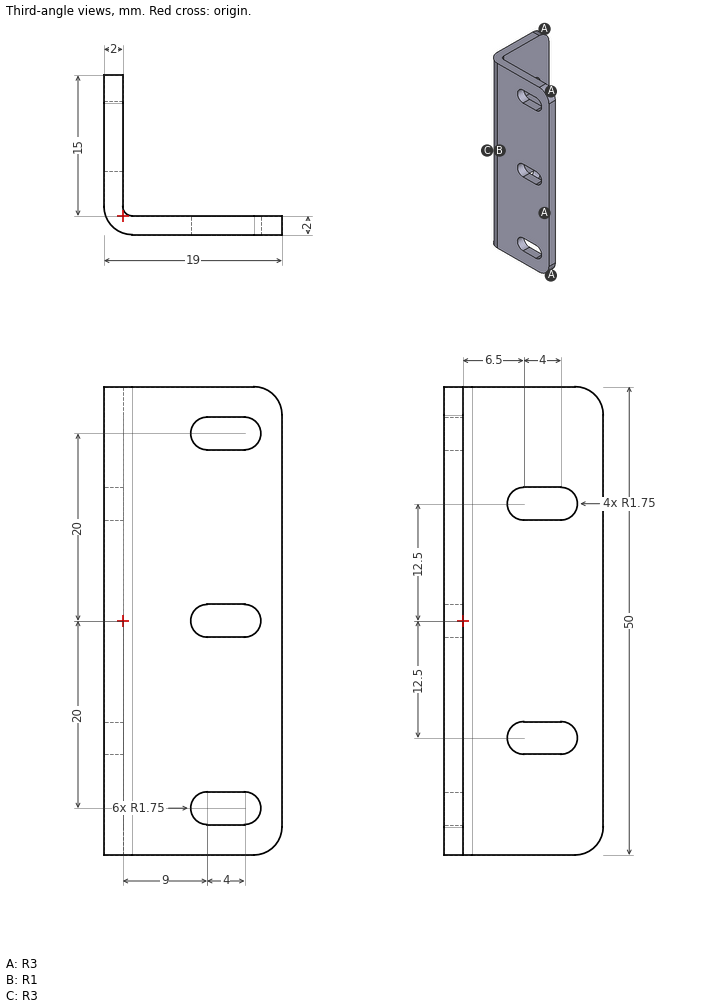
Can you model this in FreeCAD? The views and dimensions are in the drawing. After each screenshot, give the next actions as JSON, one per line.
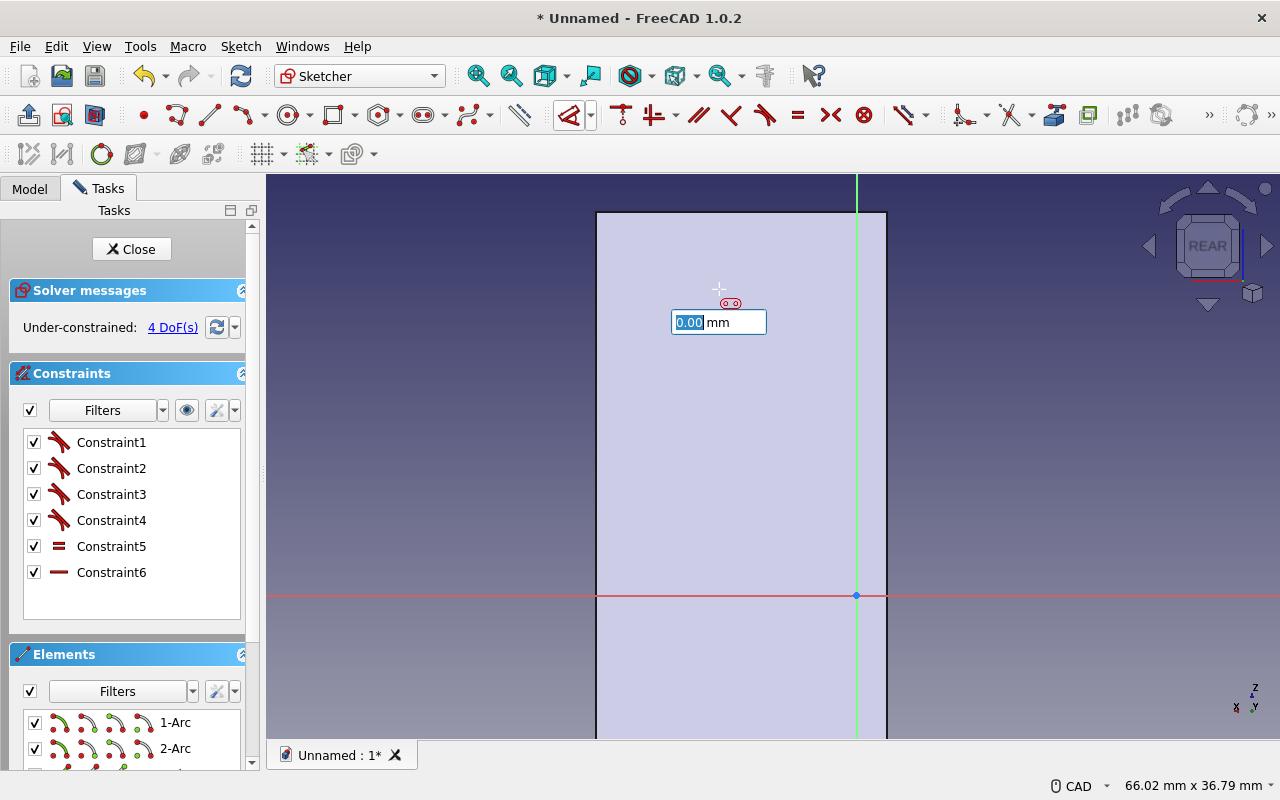
{"action": "left_click", "coordinate": [688, 262]}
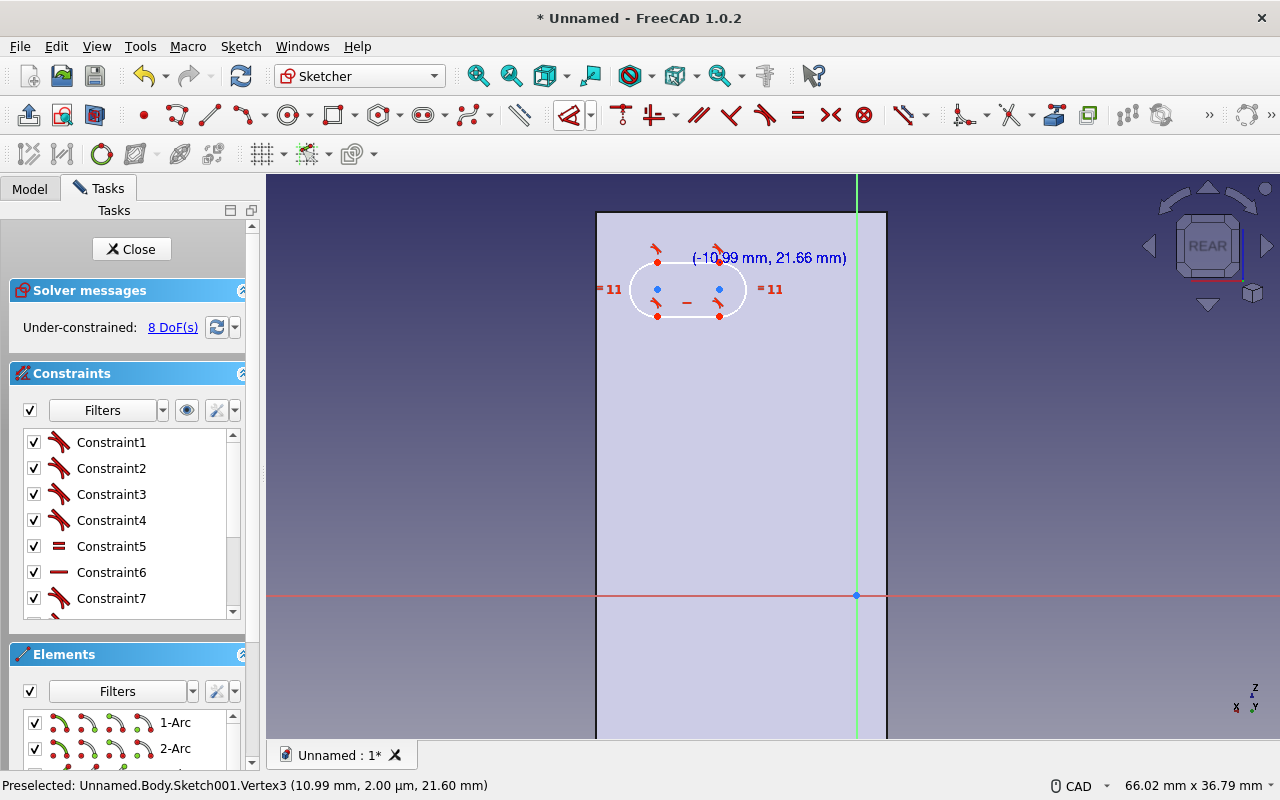
{"action": "left_click", "coordinate": [657, 596]}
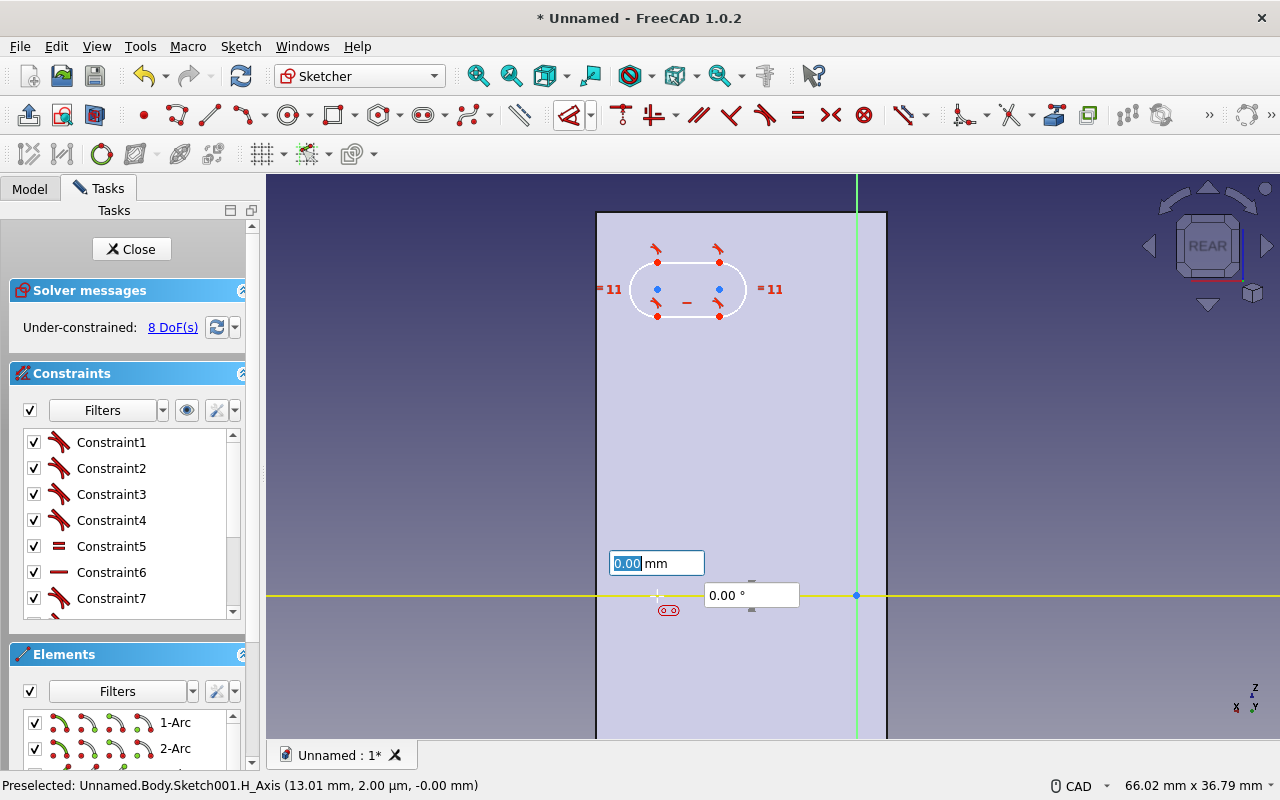
{"action": "left_click", "coordinate": [719, 587]}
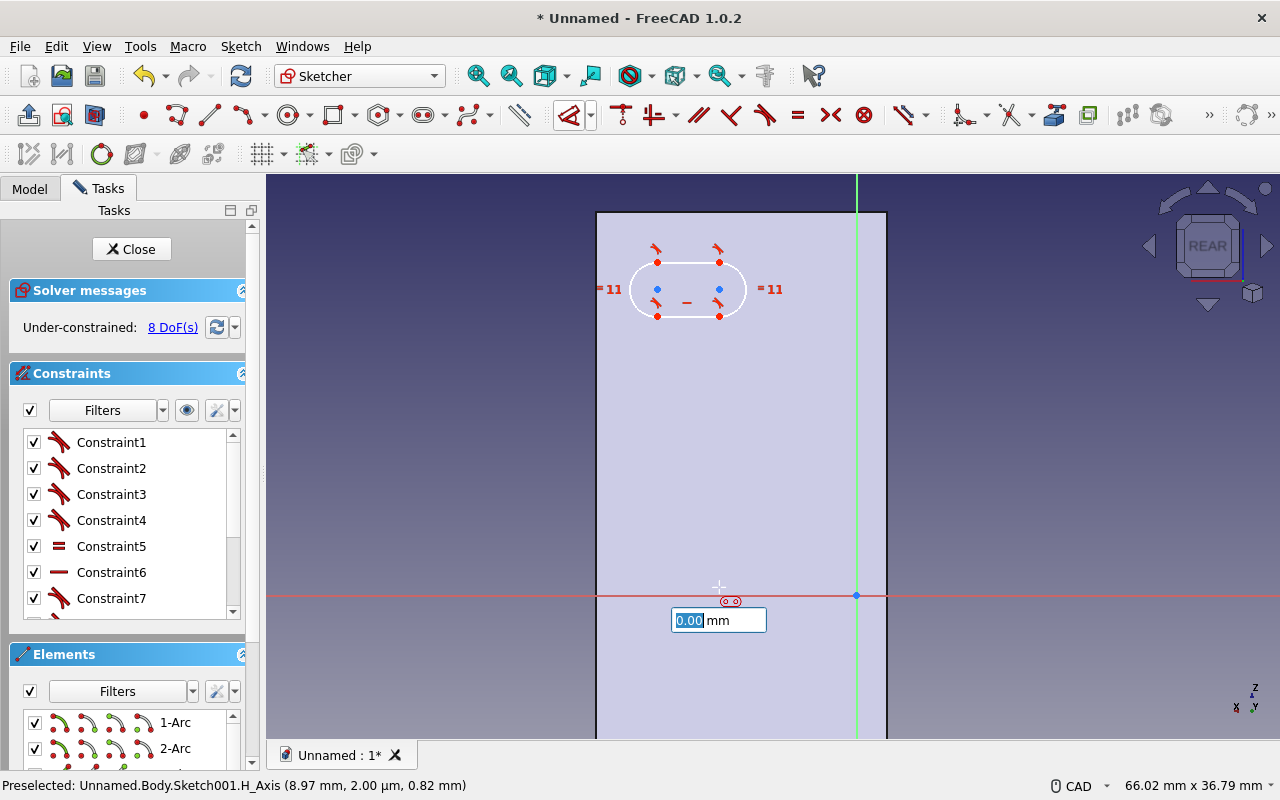
{"action": "left_click", "coordinate": [688, 623]}
{"action": "key", "text": "Escape"}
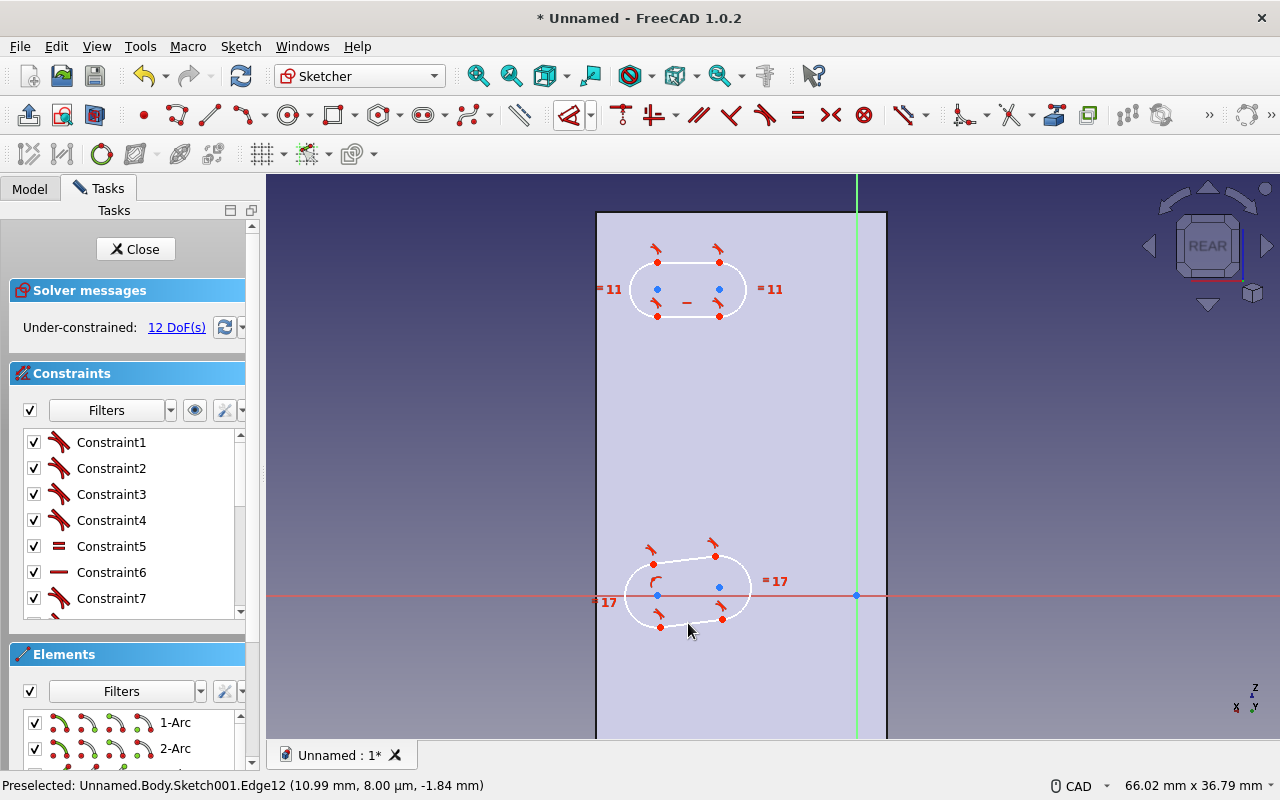
{"action": "left_click", "coordinate": [672, 562]}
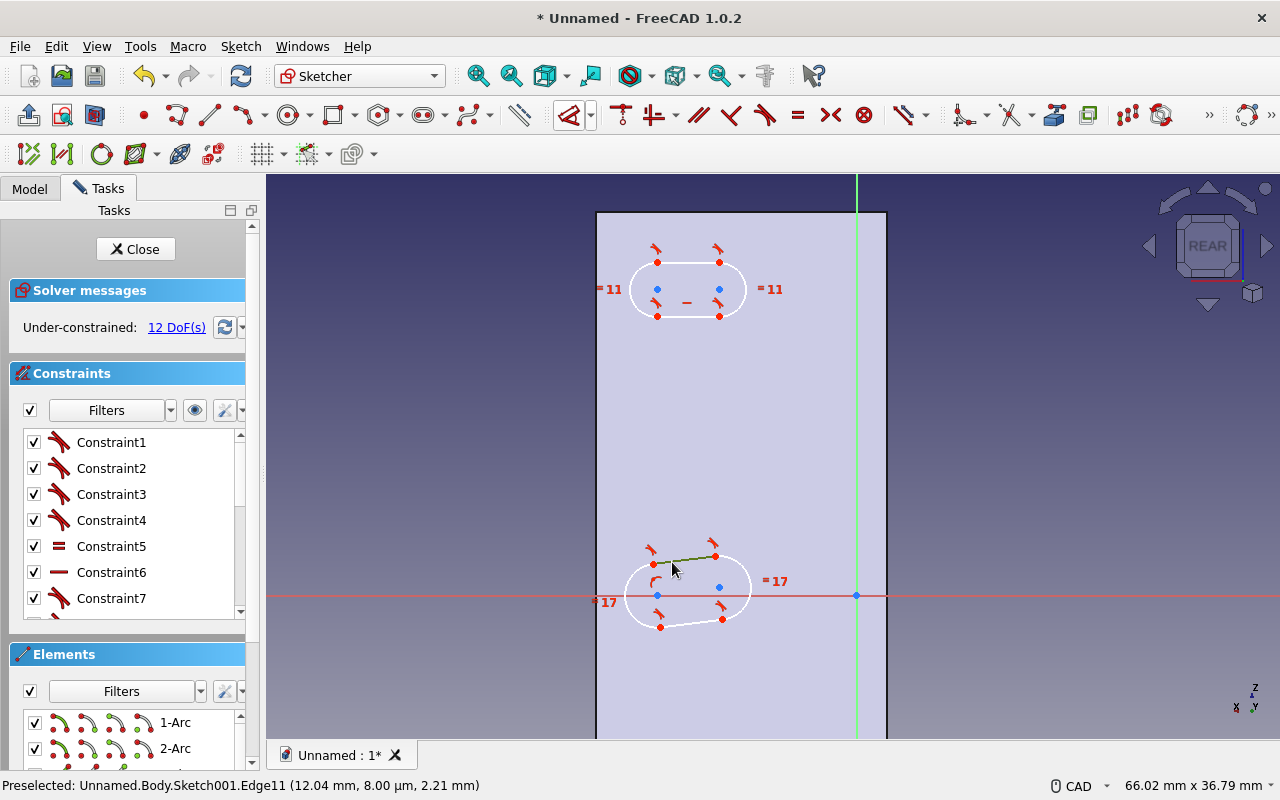
{"action": "left_click", "coordinate": [676, 116]}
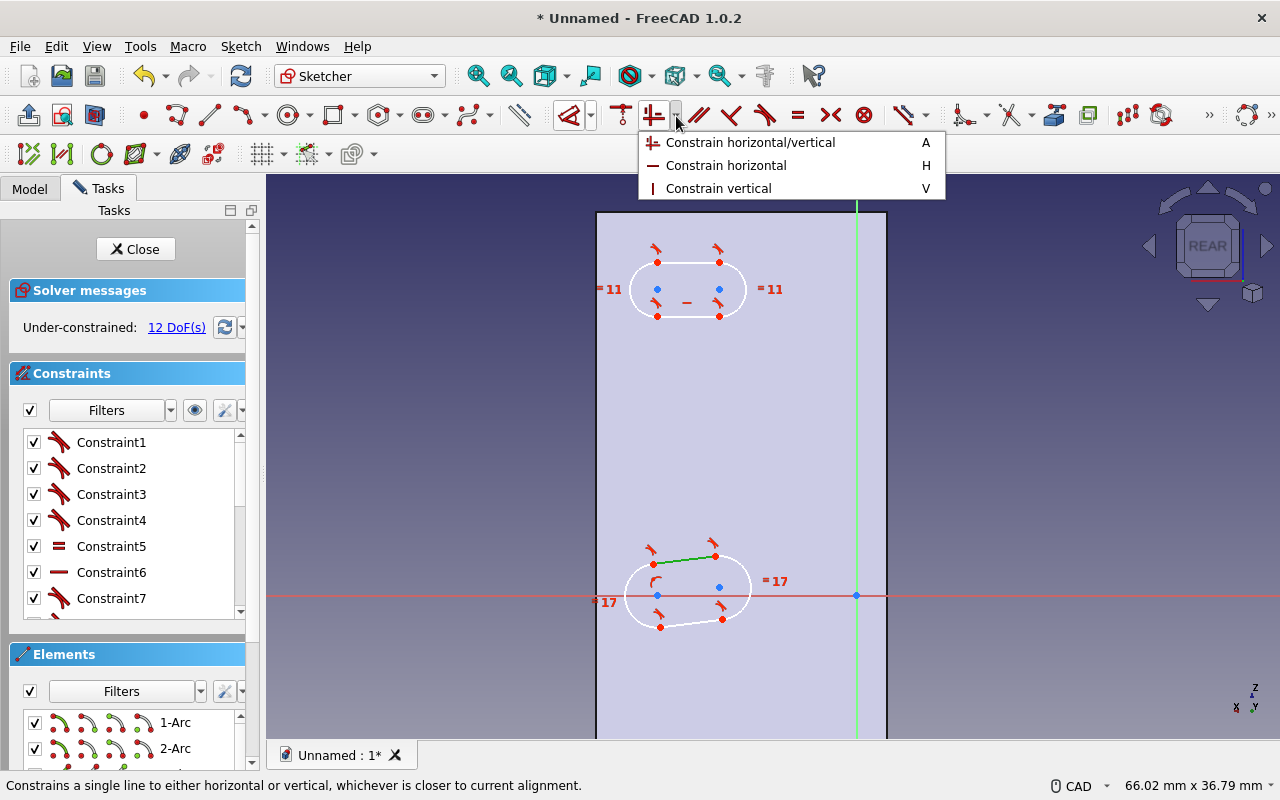
{"action": "left_click", "coordinate": [792, 166]}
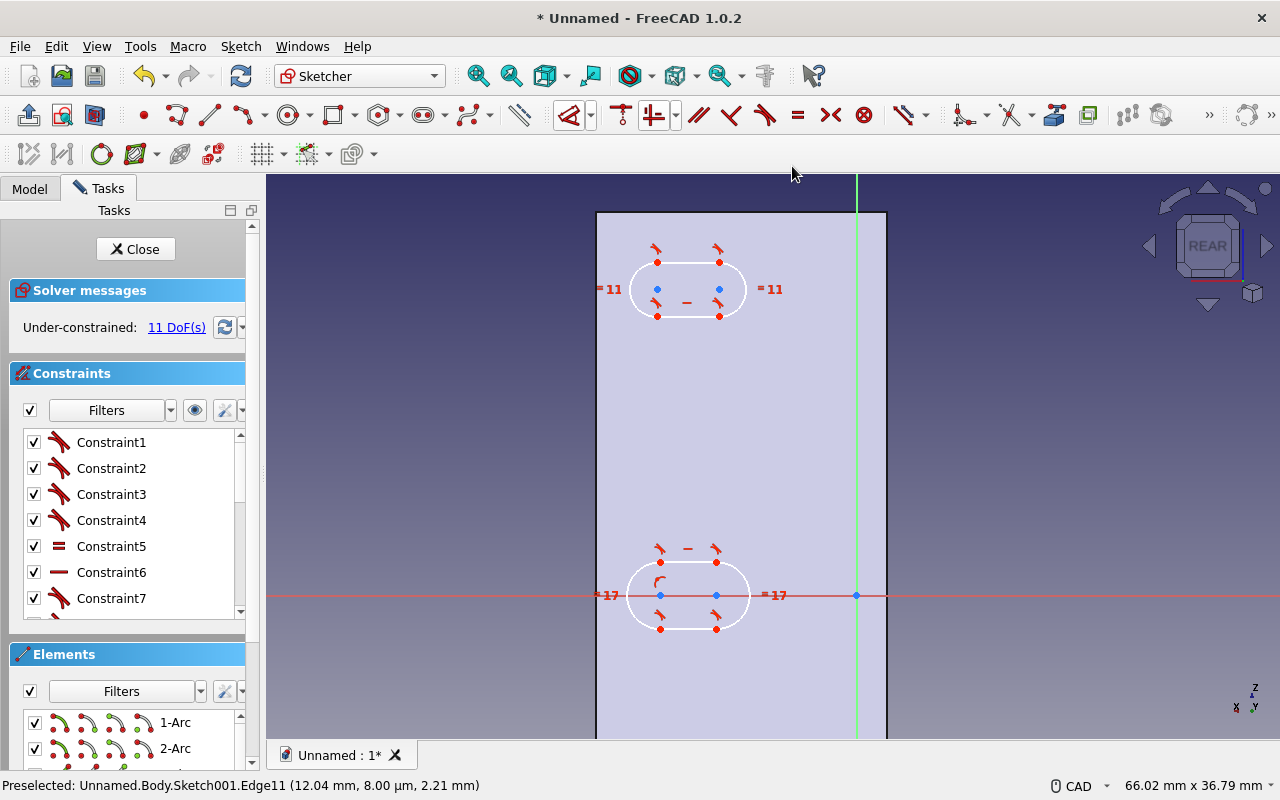
{"action": "scroll", "coordinate": [657, 287], "scroll_direction": "down", "scroll_amount": 3}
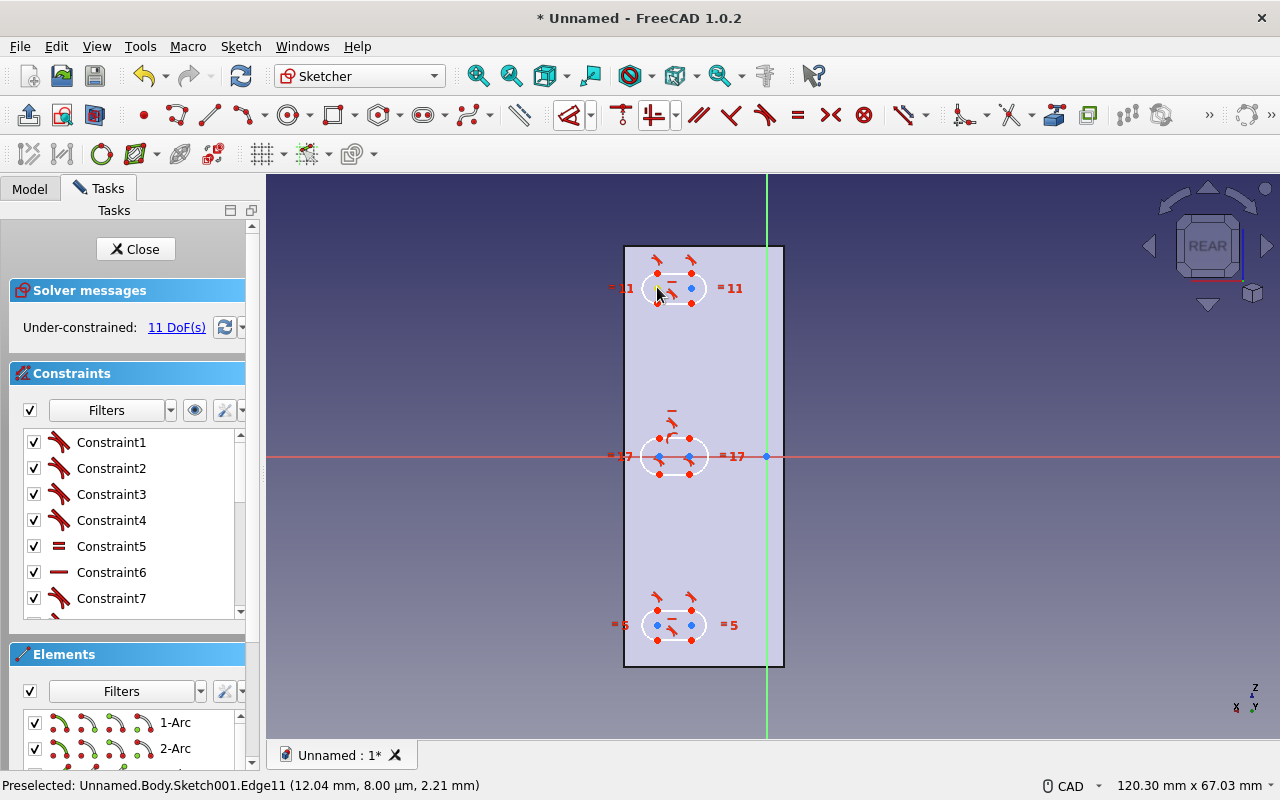
{"action": "left_click", "coordinate": [645, 617]}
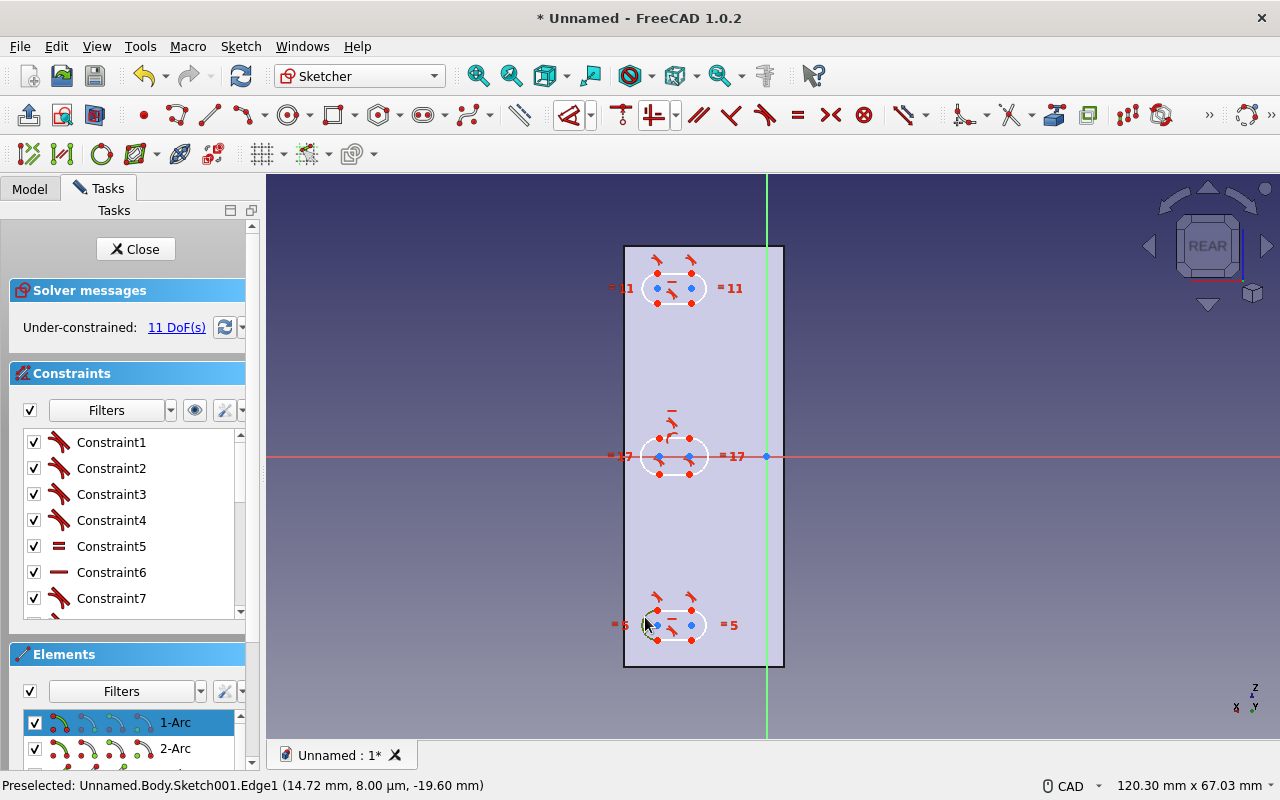
{"action": "left_click", "coordinate": [645, 280]}